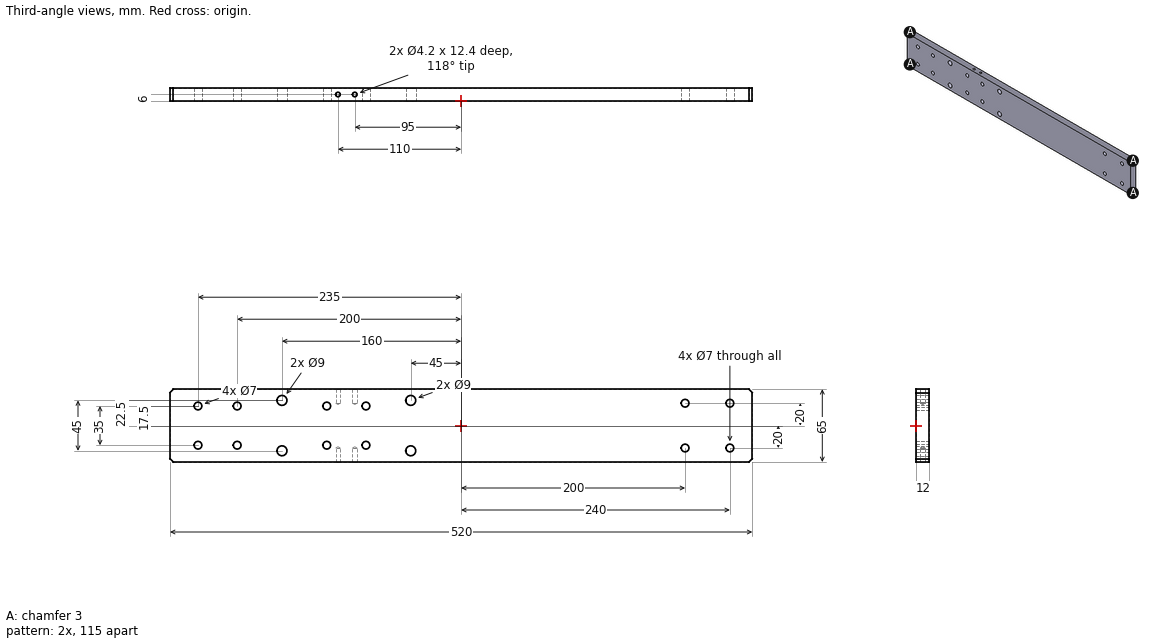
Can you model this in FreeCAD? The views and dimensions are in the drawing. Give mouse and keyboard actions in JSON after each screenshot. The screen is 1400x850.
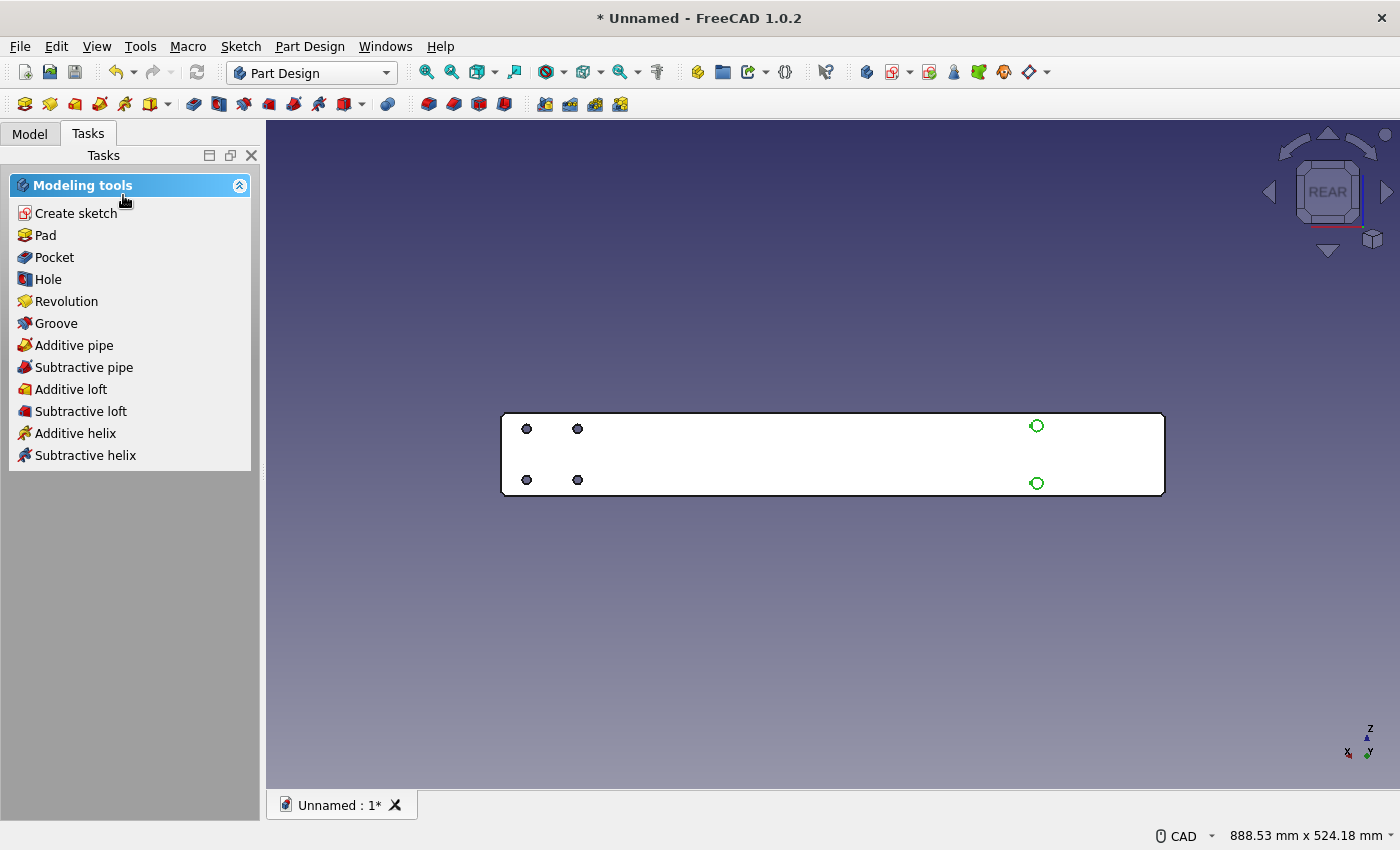
{"action": "left_click", "coordinate": [194, 104]}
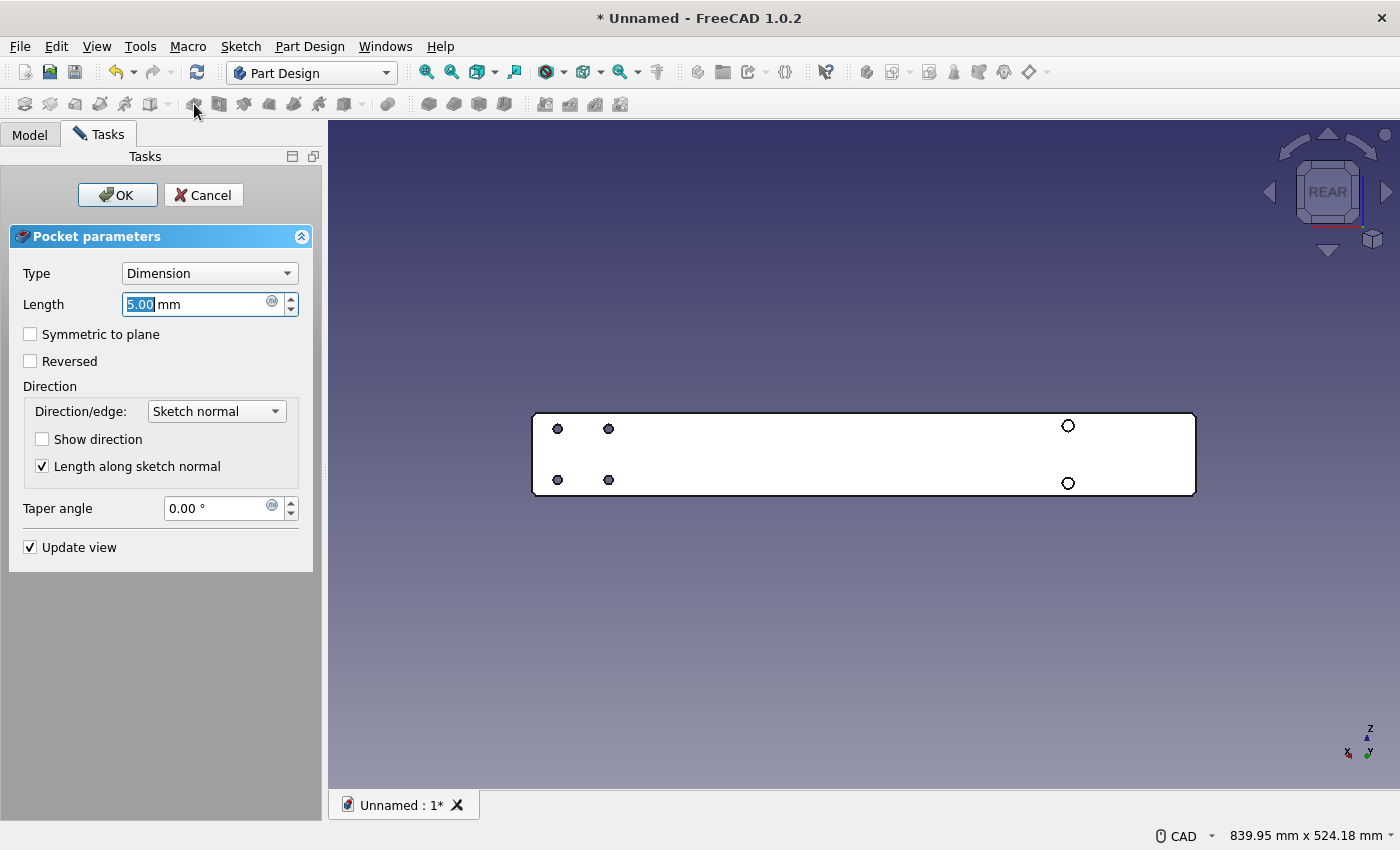
{"action": "left_click", "coordinate": [210, 274]}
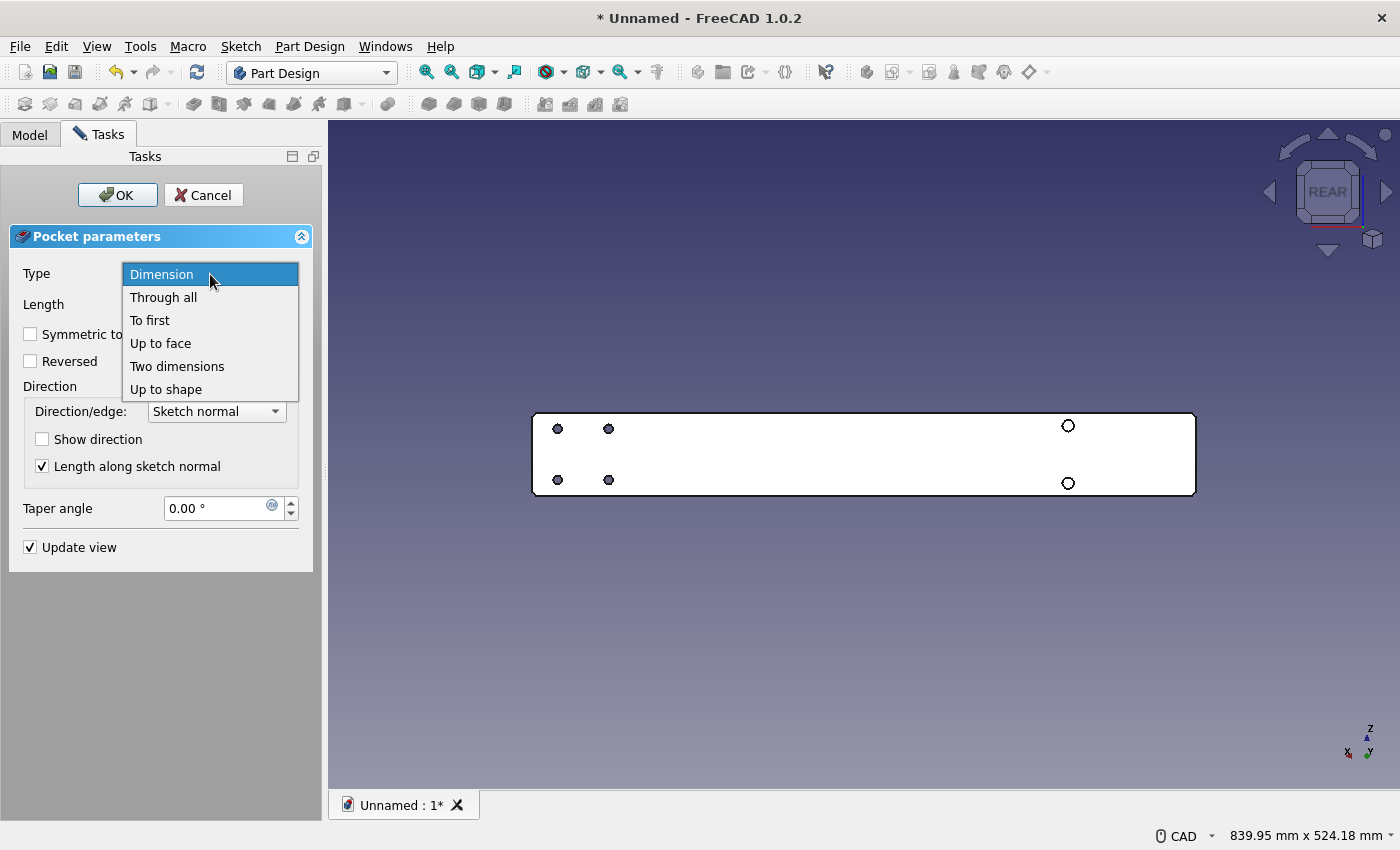
{"action": "left_click", "coordinate": [208, 298]}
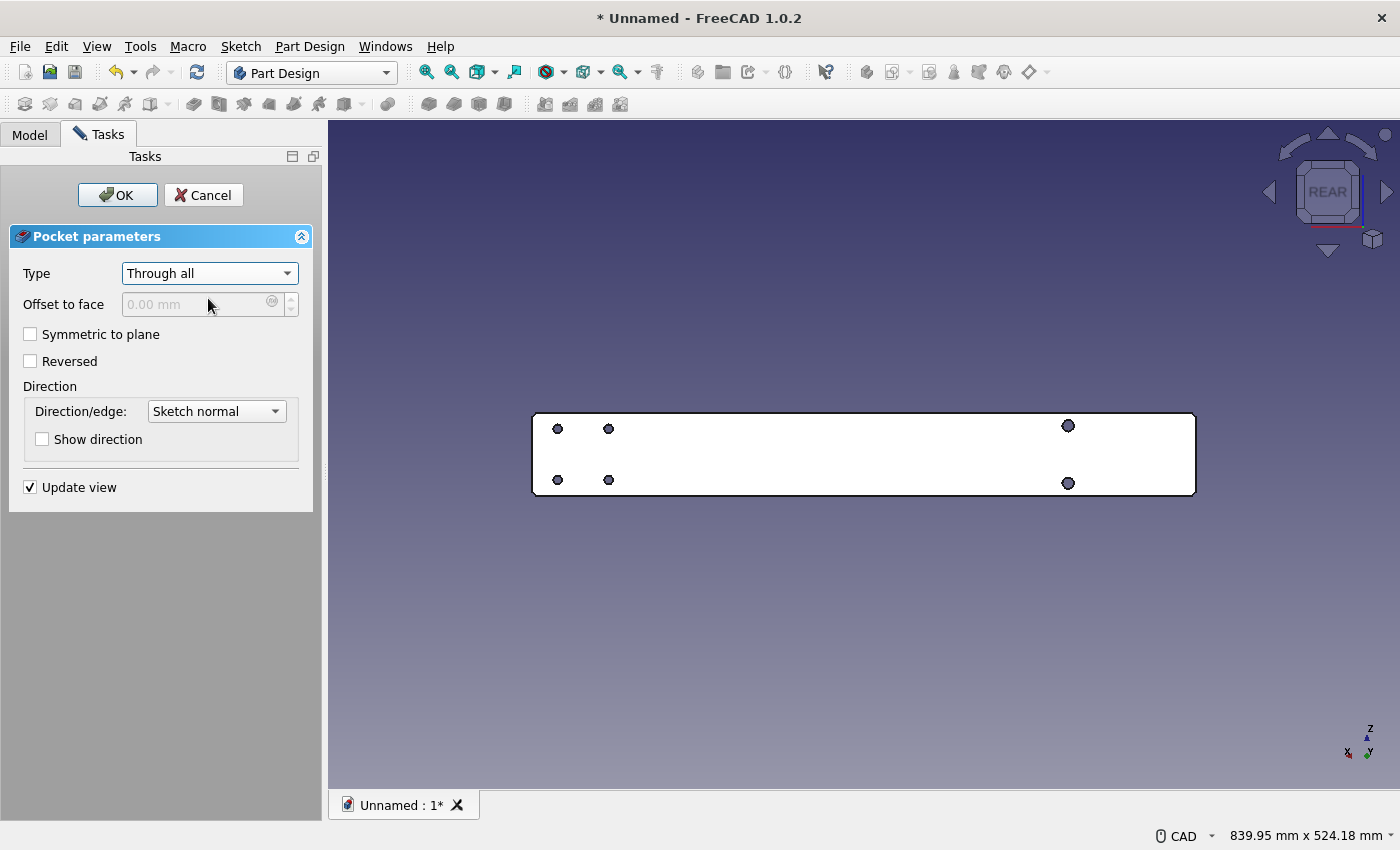
{"action": "left_click", "coordinate": [118, 195]}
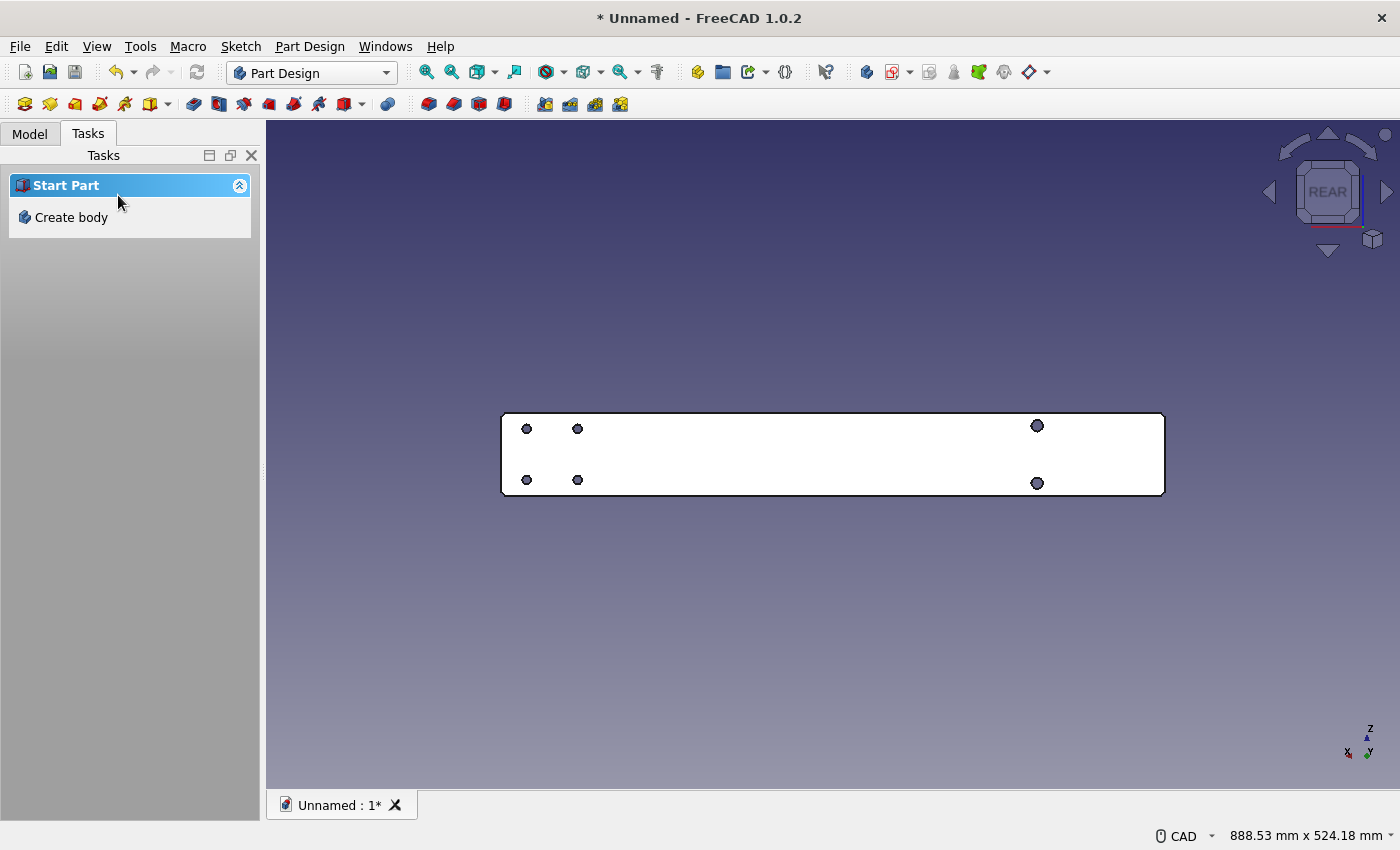
{"action": "left_click", "coordinate": [643, 454]}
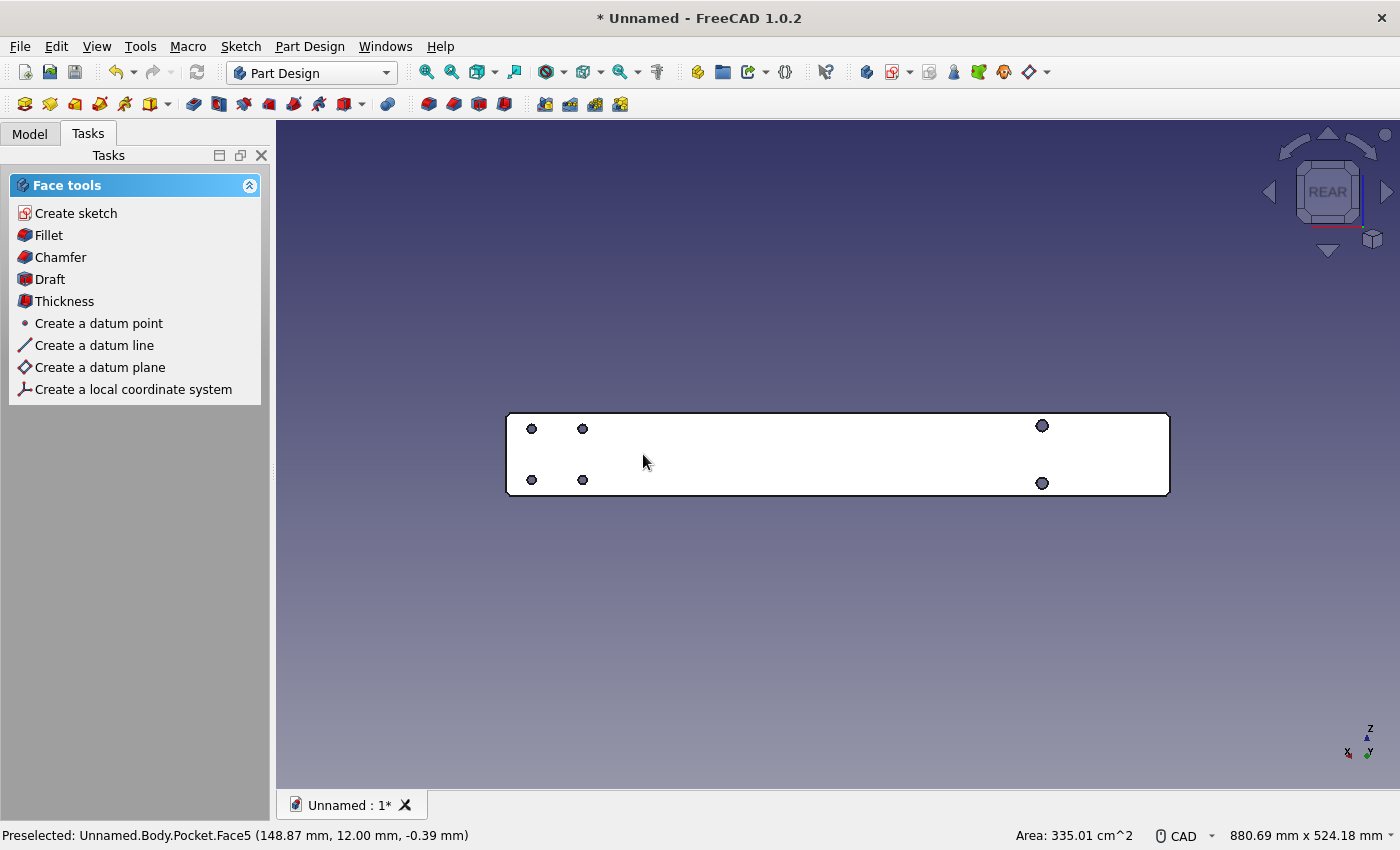
{"action": "left_click", "coordinate": [892, 72]}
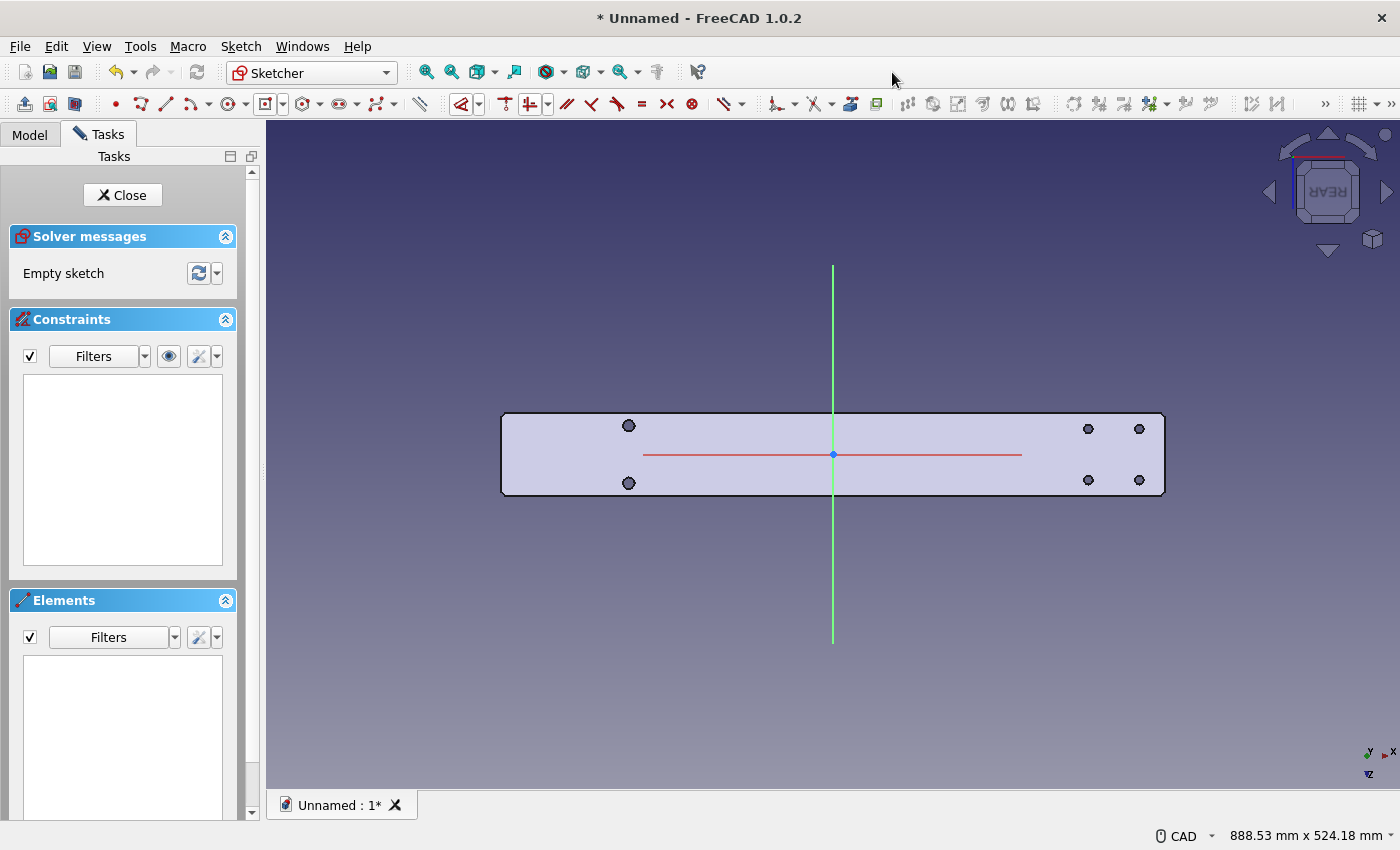
{"action": "scroll", "coordinate": [523, 454], "scroll_direction": "up", "scroll_amount": 10}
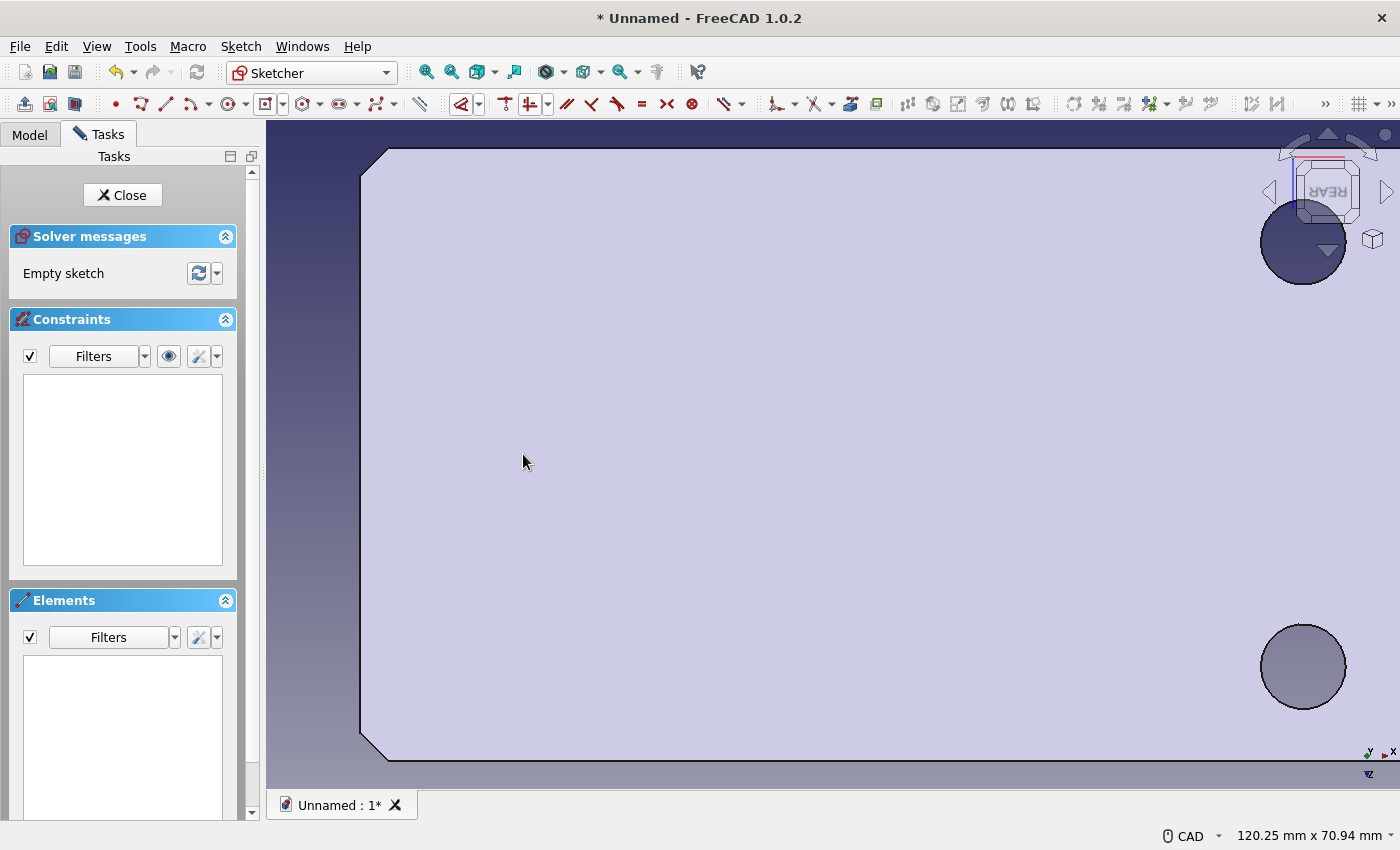
{"action": "left_click", "coordinate": [228, 104]}